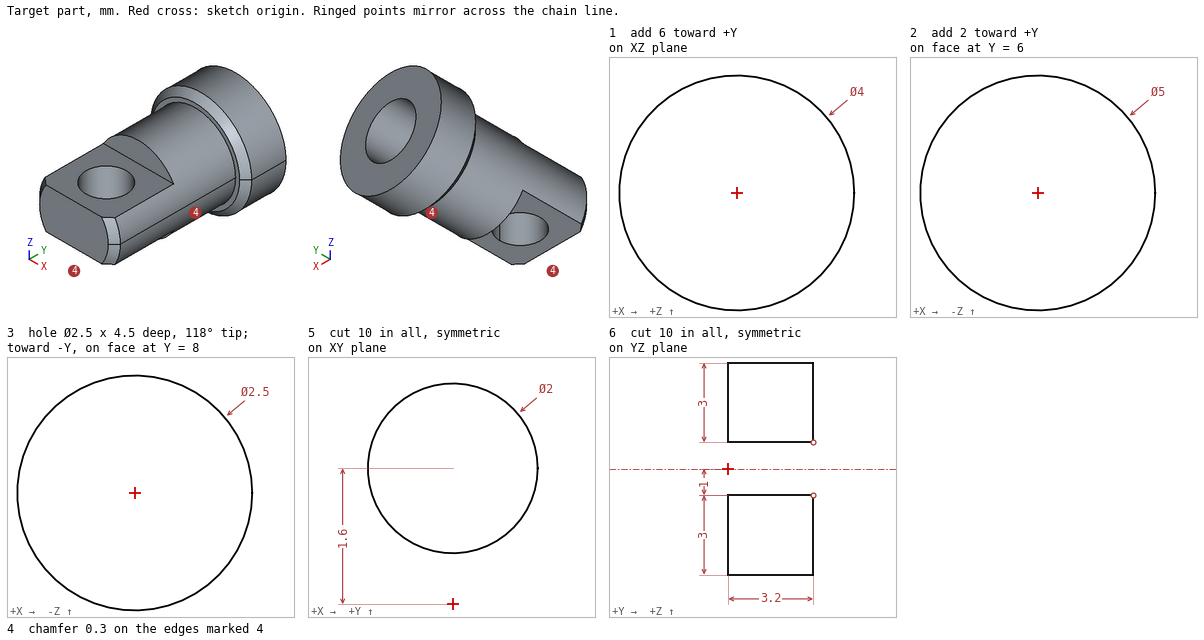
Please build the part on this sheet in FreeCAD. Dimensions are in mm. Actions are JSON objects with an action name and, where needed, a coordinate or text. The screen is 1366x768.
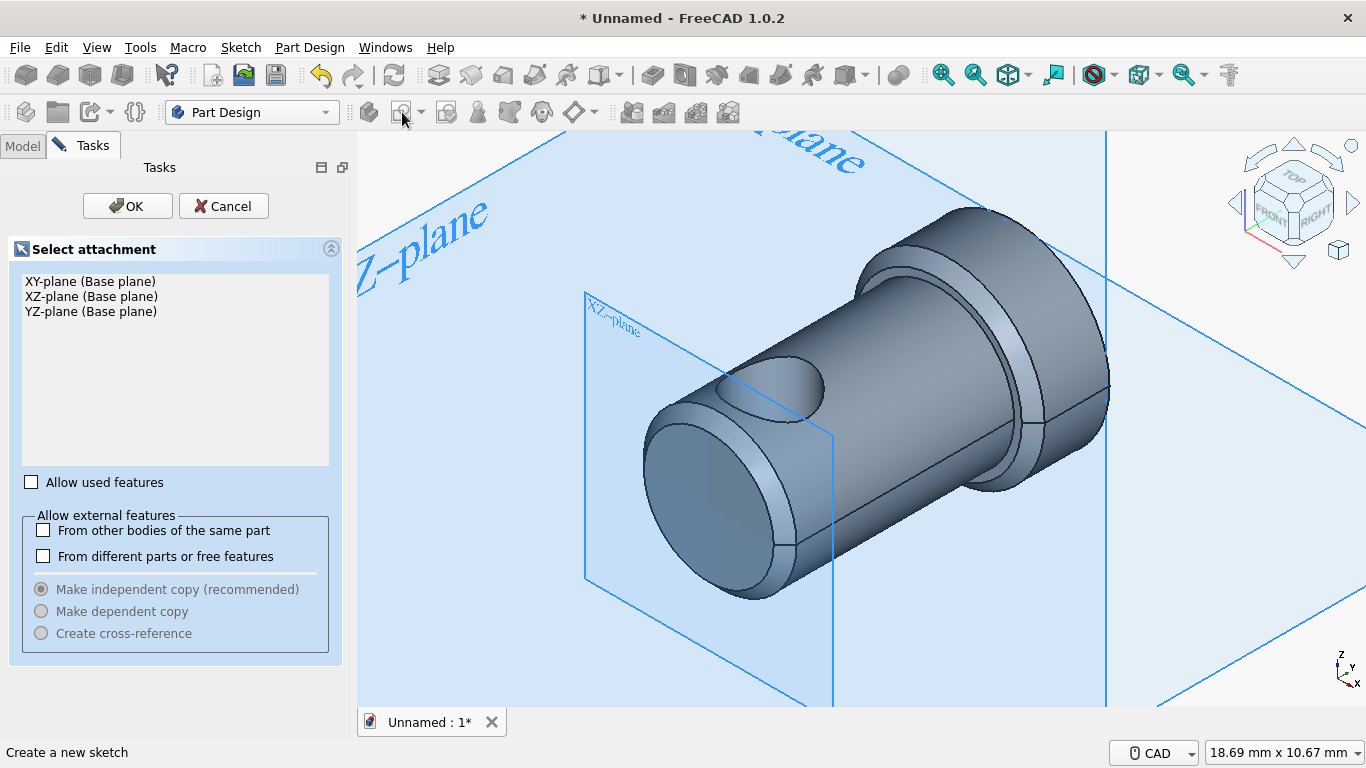
{"action": "left_click", "coordinate": [82, 312]}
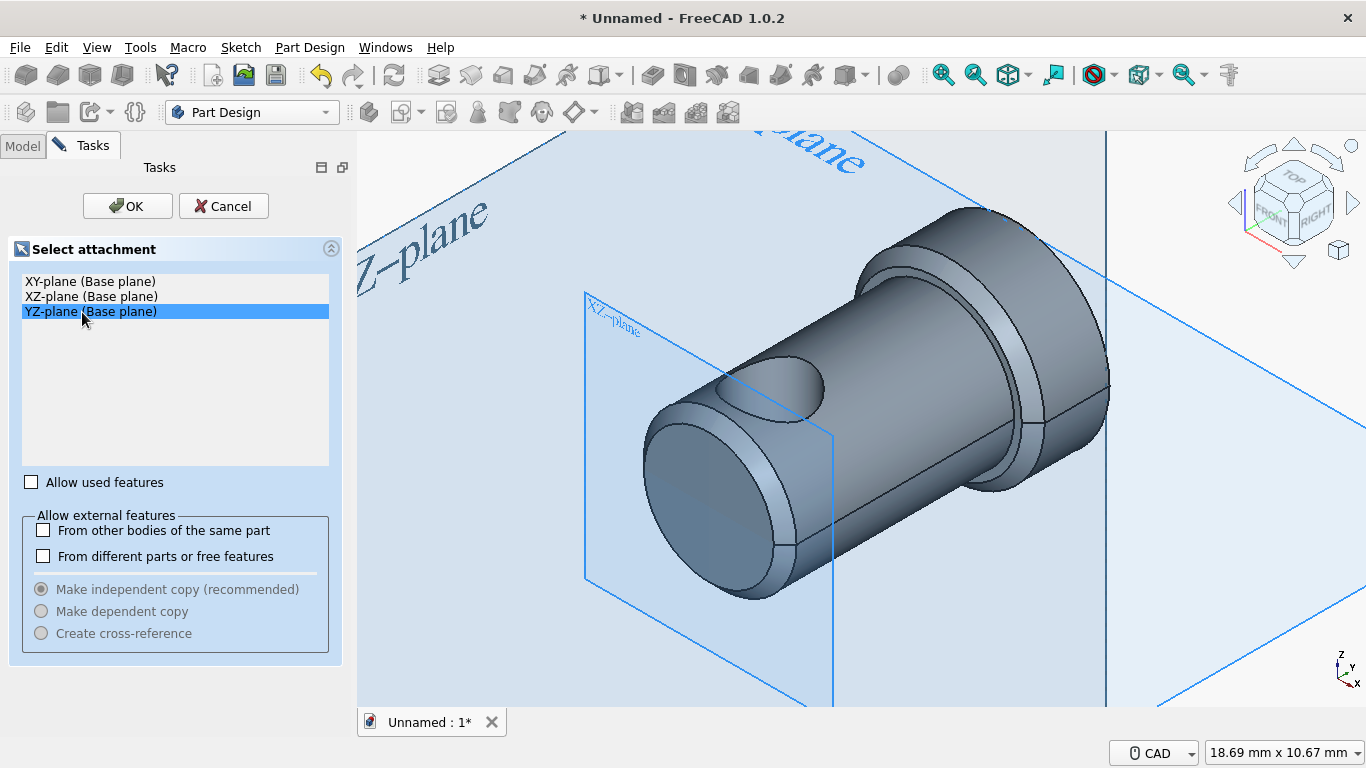
{"action": "left_click", "coordinate": [128, 206]}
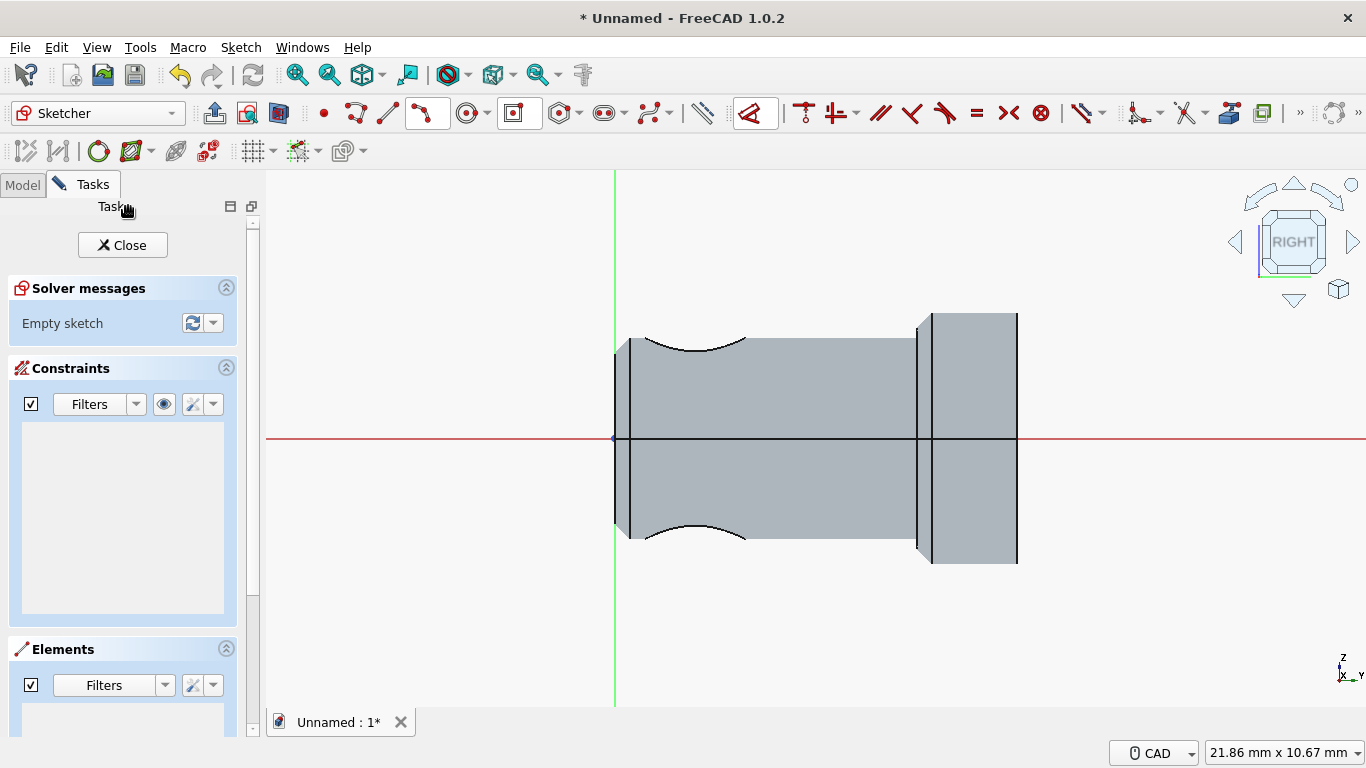
{"action": "key", "text": "q s"}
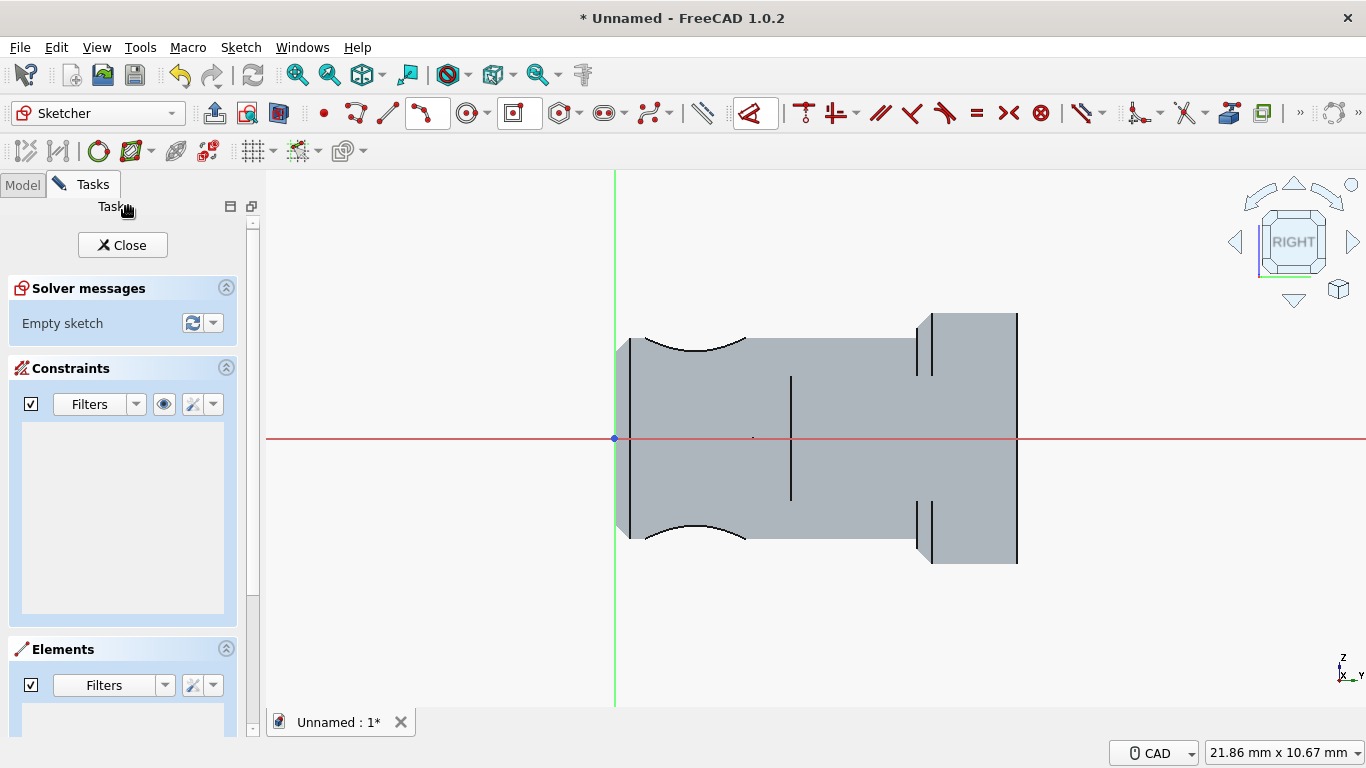
{"action": "key", "text": "g r"}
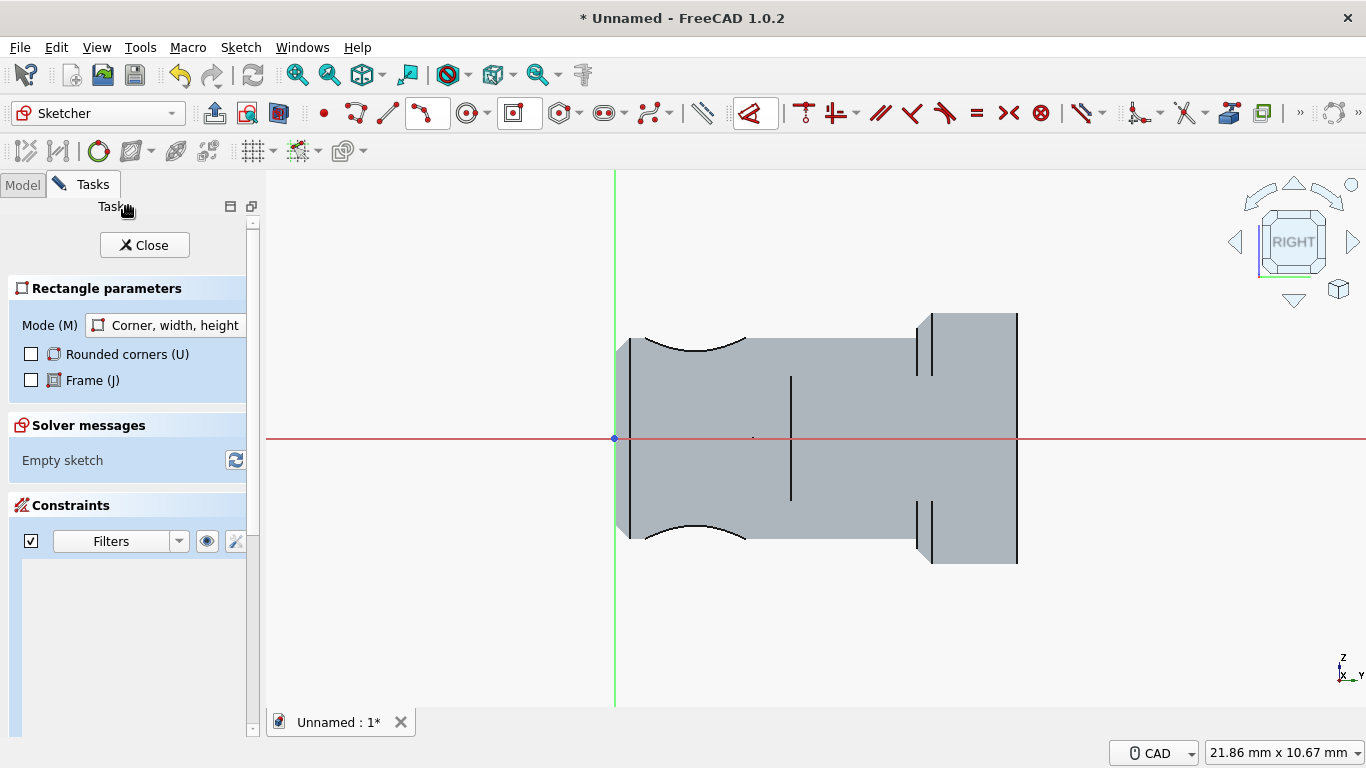
{"action": "left_click", "coordinate": [615, 489]}
{"action": "left_click", "coordinate": [776, 640]}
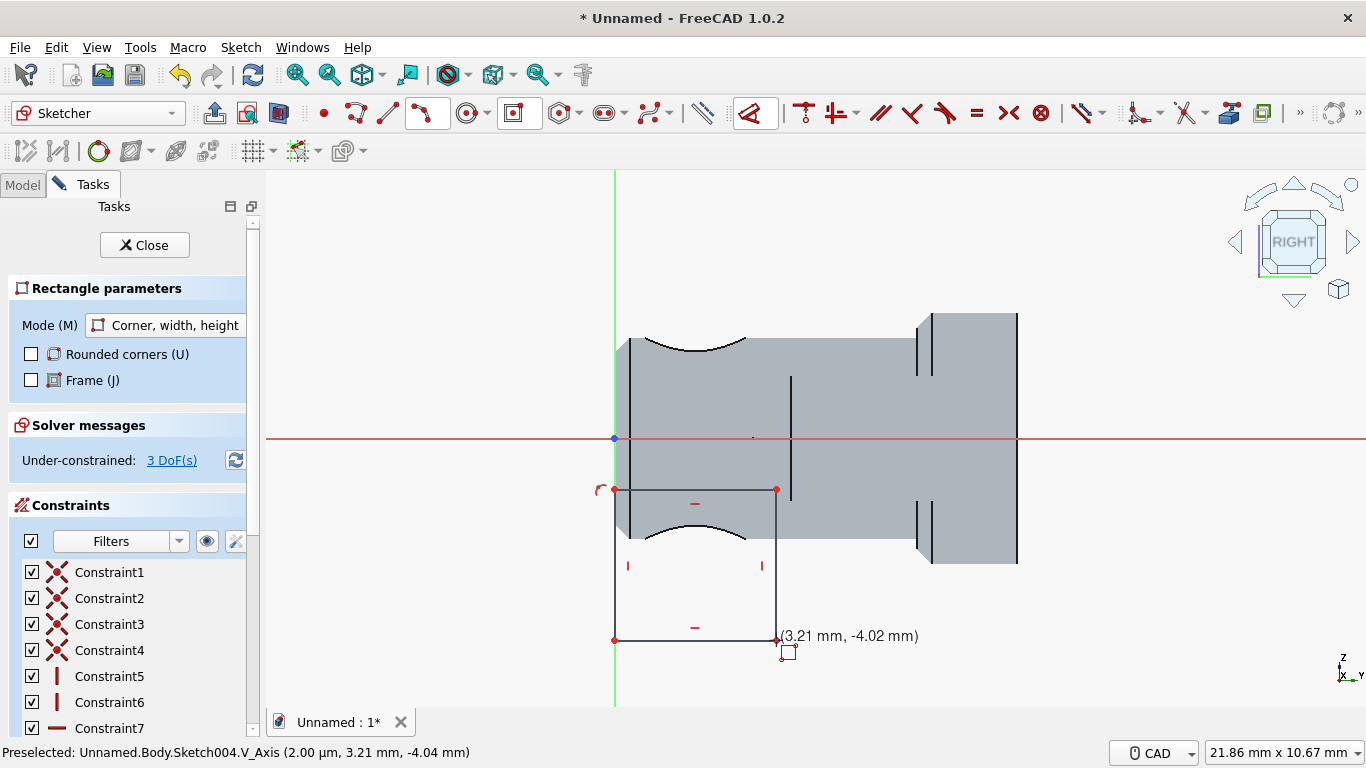
{"action": "left_click", "coordinate": [615, 237]}
{"action": "left_click", "coordinate": [776, 388]}
{"action": "key", "text": "Escape"}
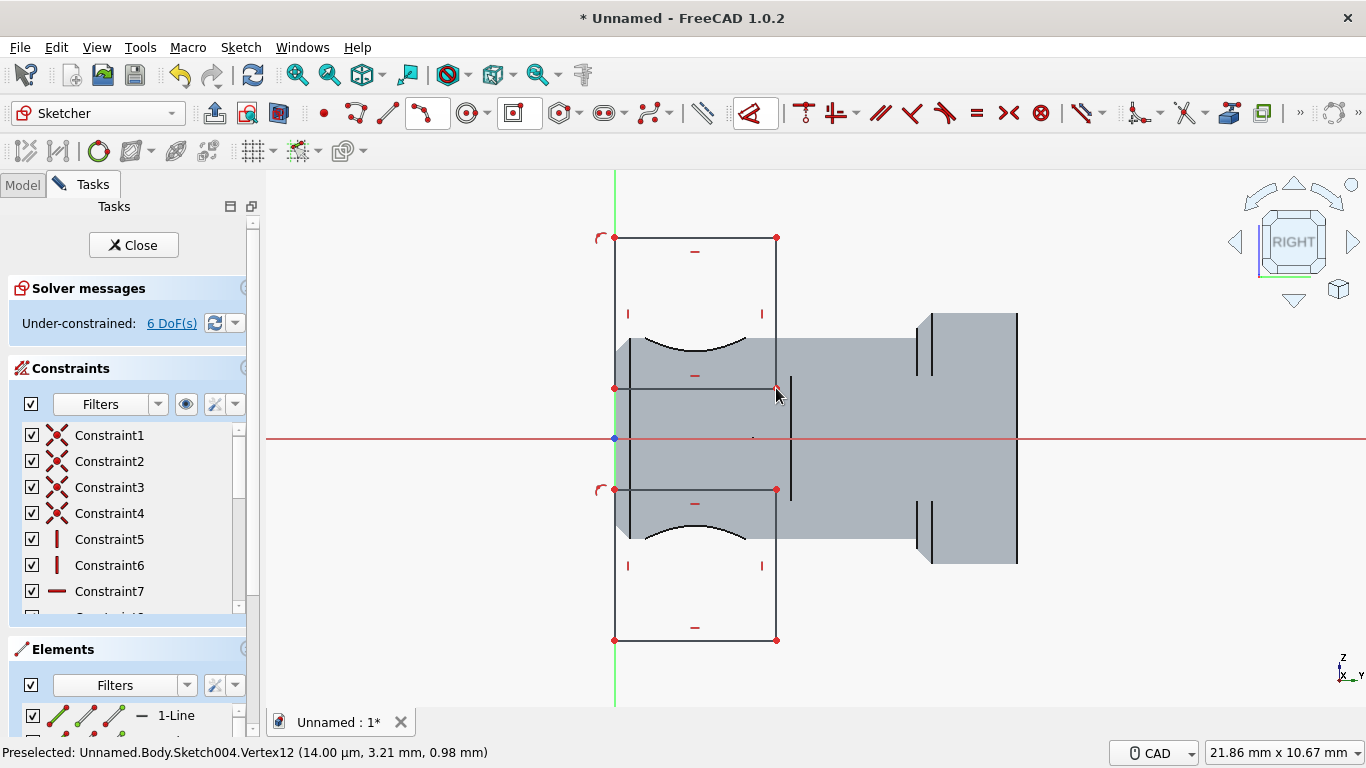
{"action": "left_click", "coordinate": [776, 490]}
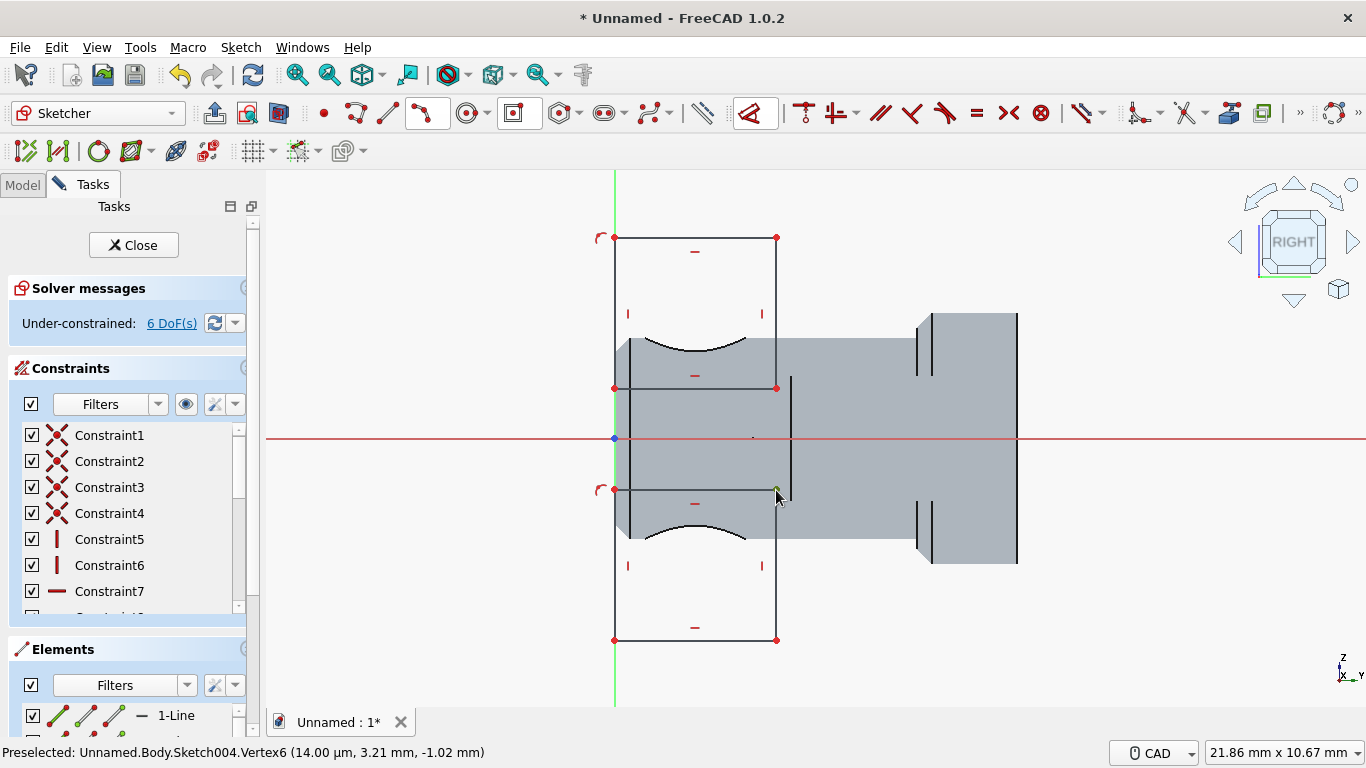
{"action": "left_click", "coordinate": [776, 389]}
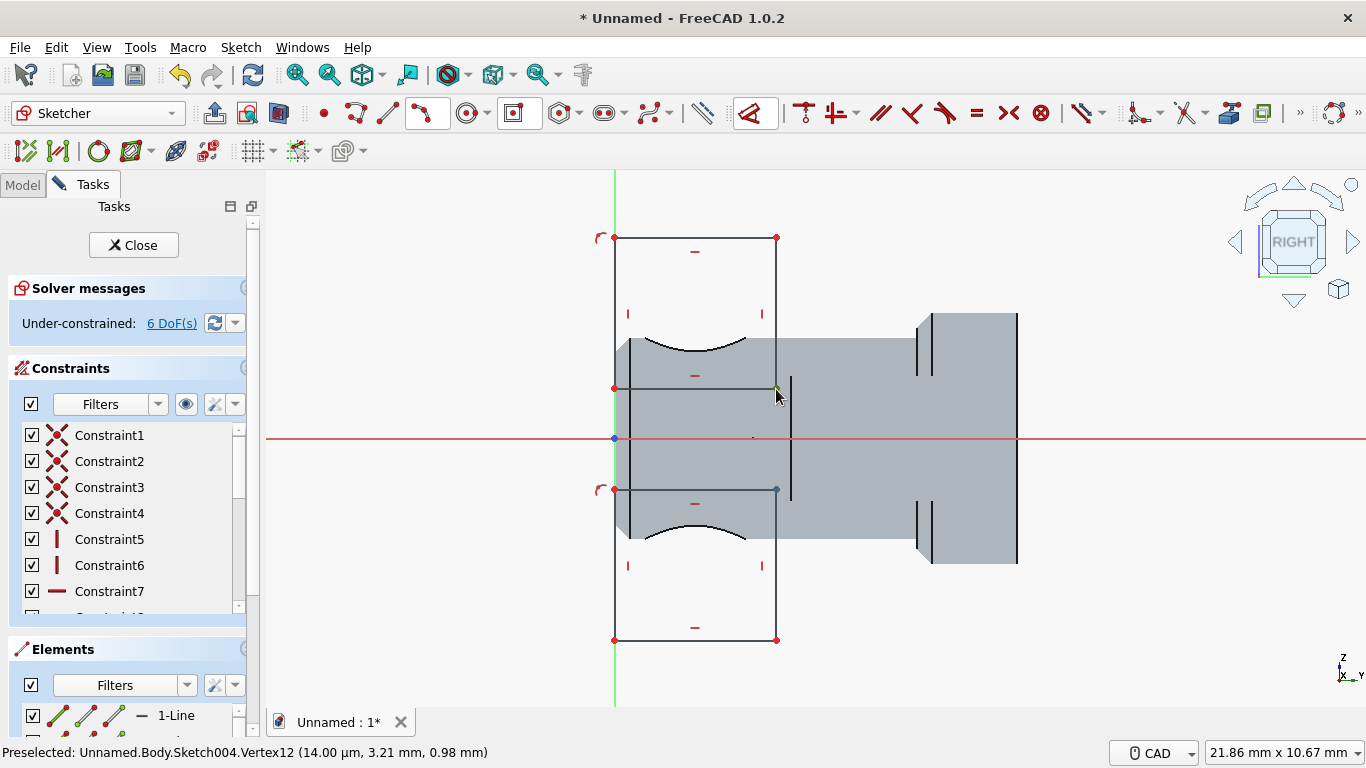
{"action": "left_click", "coordinate": [359, 439]}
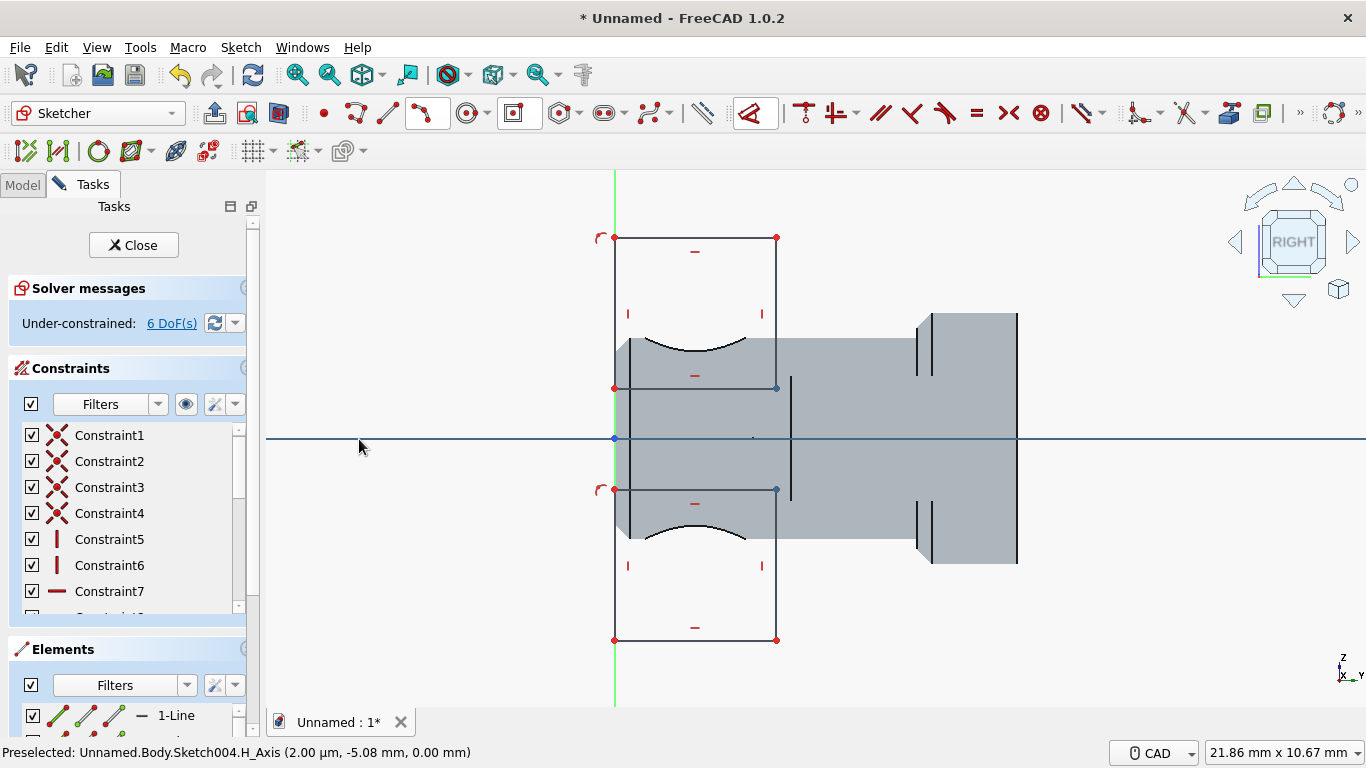
{"action": "key", "text": "s"}